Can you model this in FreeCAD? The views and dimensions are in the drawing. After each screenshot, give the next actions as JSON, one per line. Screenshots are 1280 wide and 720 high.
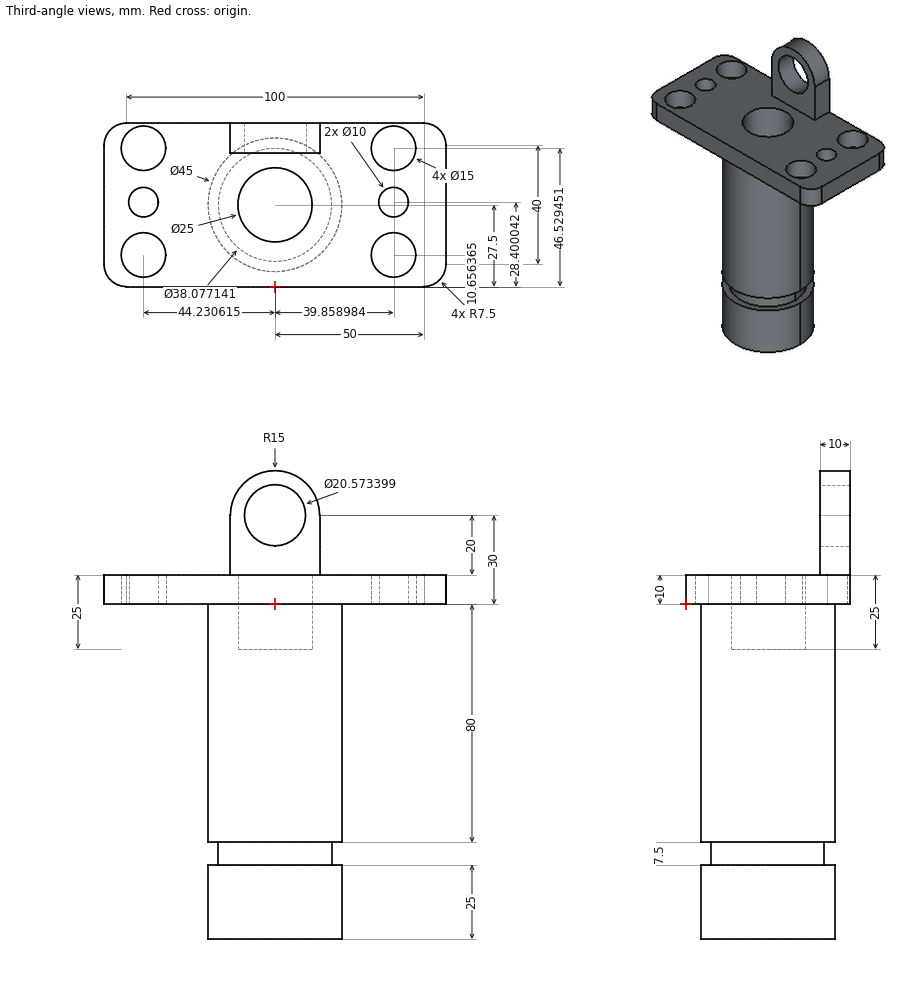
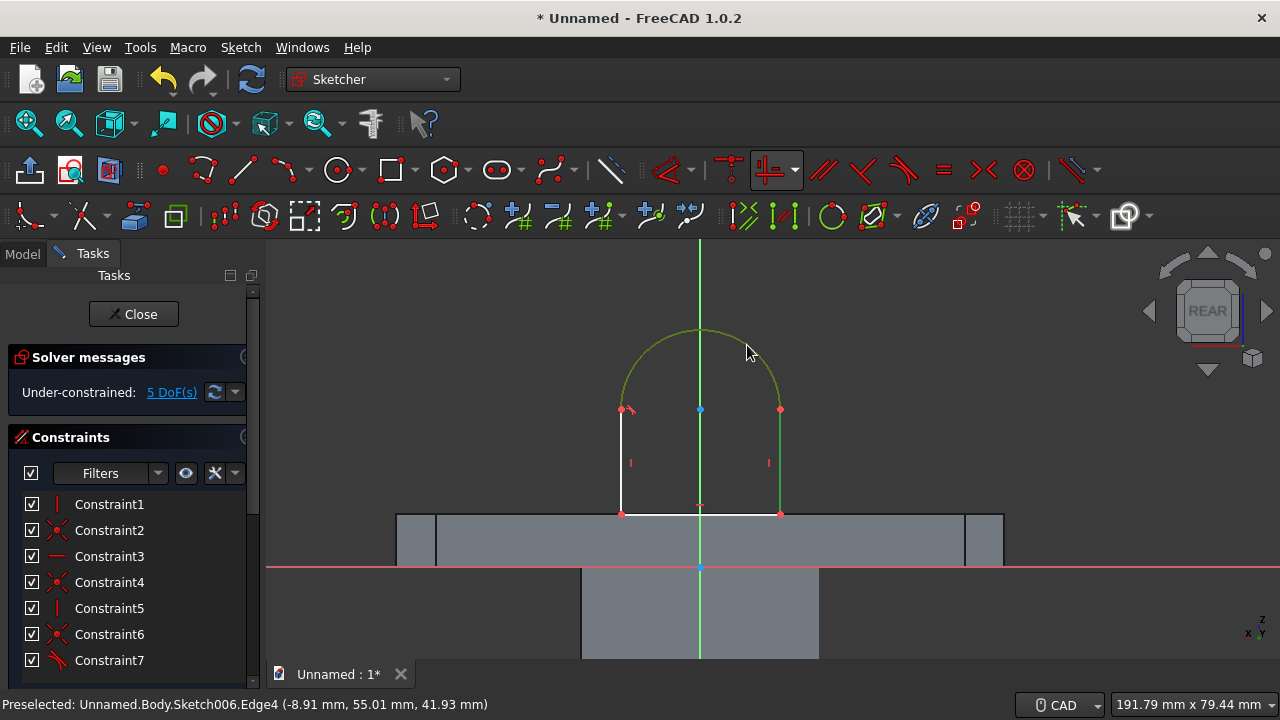
{"action": "left_click", "coordinate": [904, 170]}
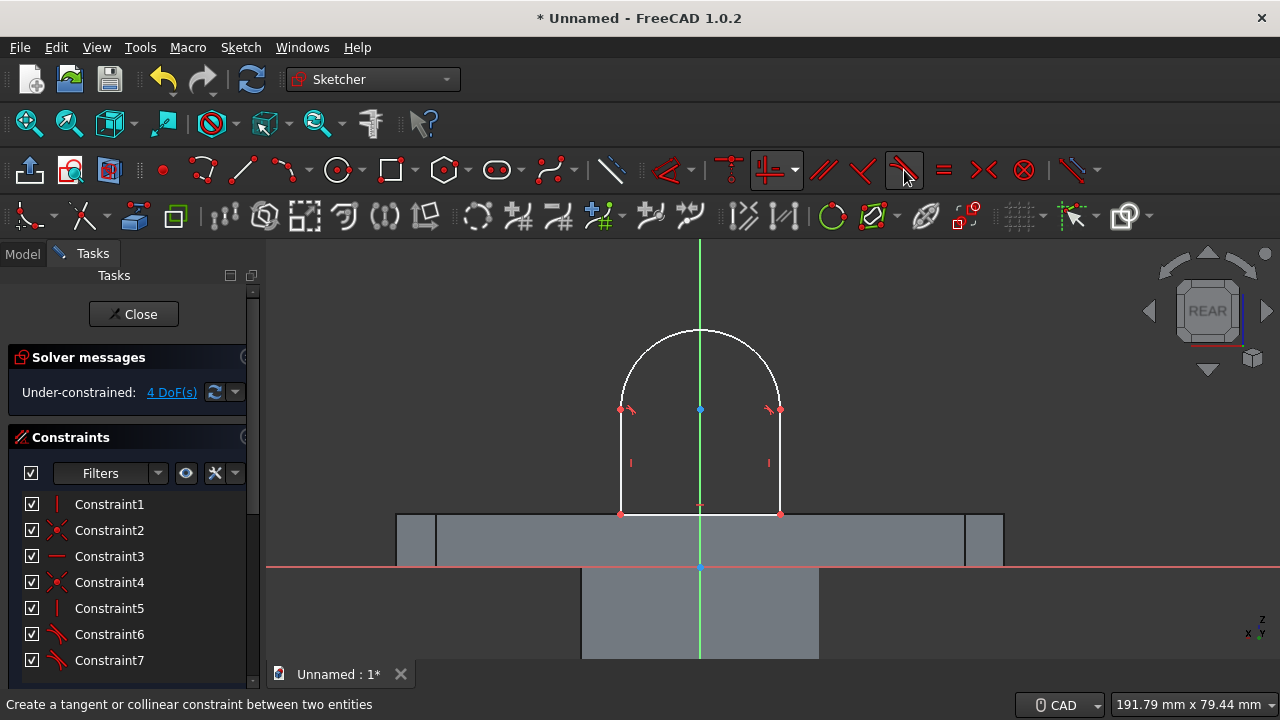
{"action": "left_click", "coordinate": [700, 410]}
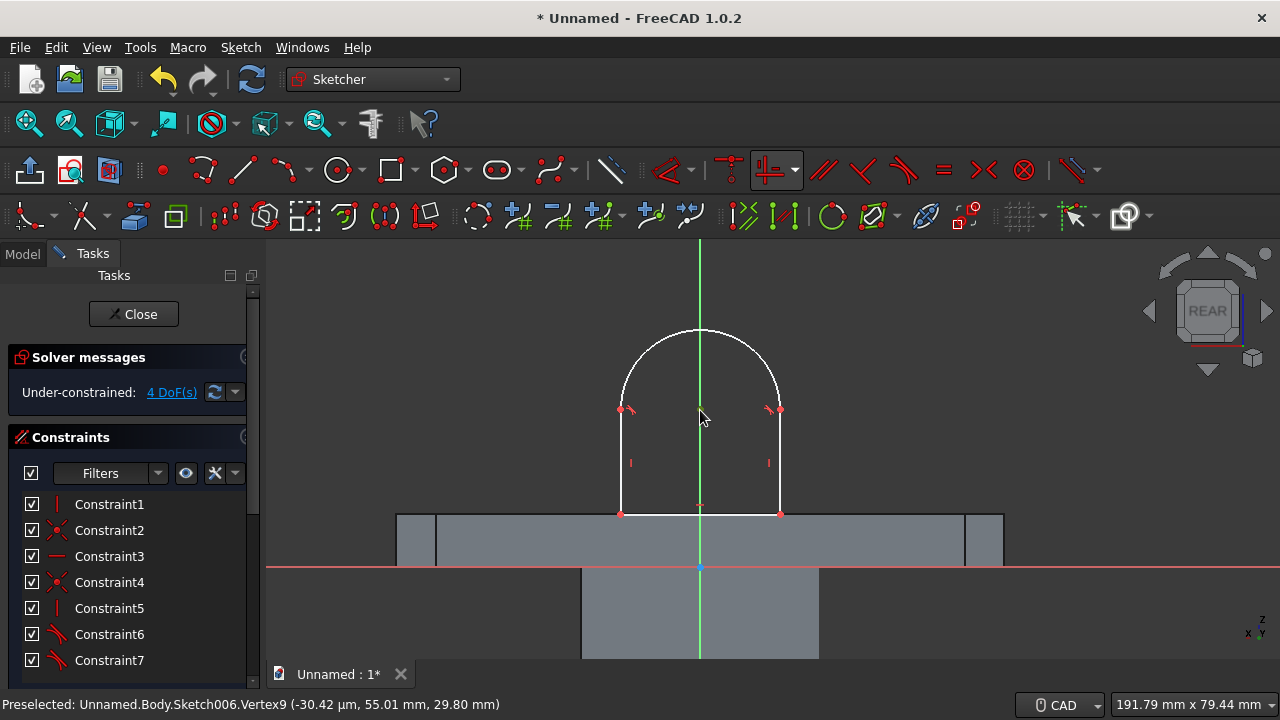
{"action": "left_click", "coordinate": [700, 605]}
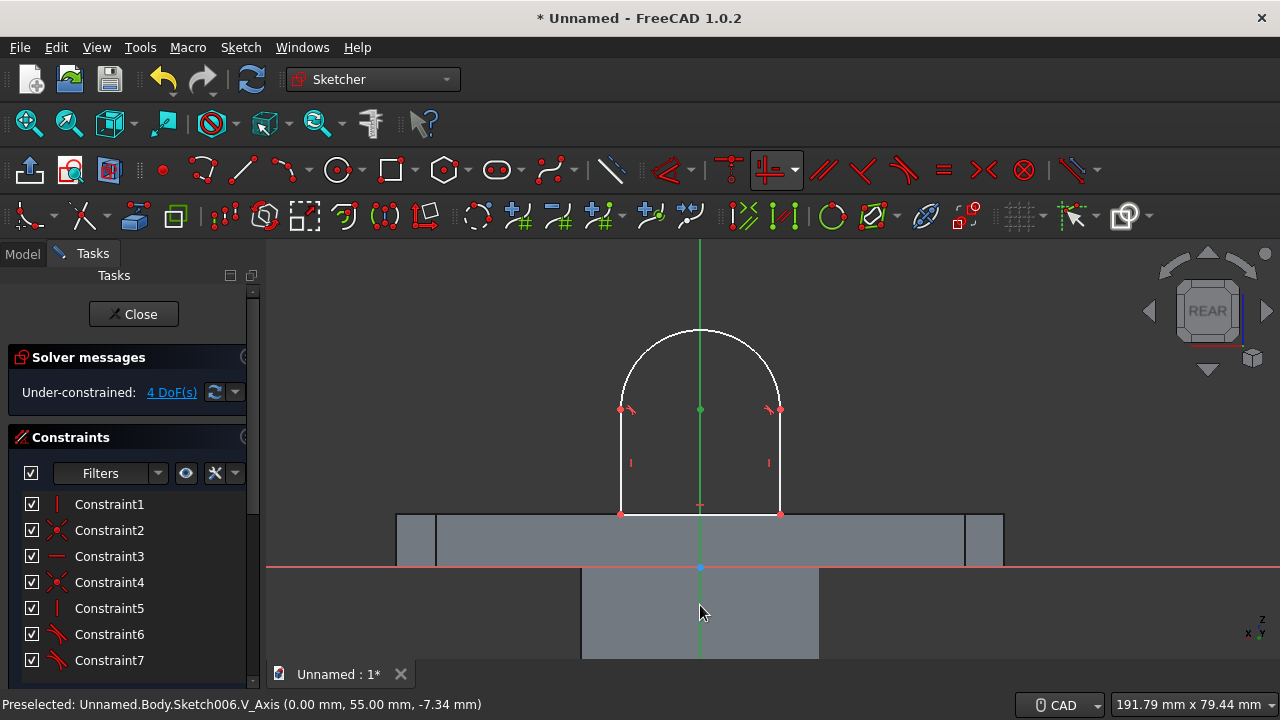
{"action": "left_click", "coordinate": [730, 170]}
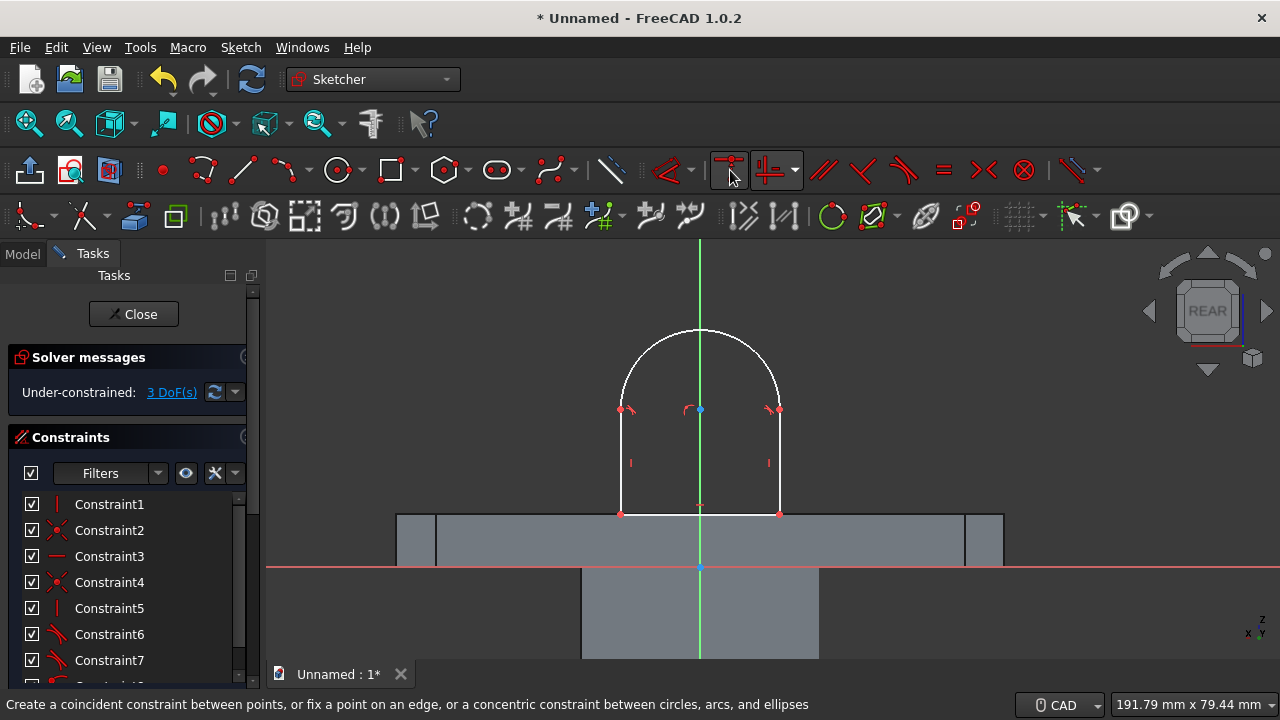
{"action": "left_click", "coordinate": [666, 170]}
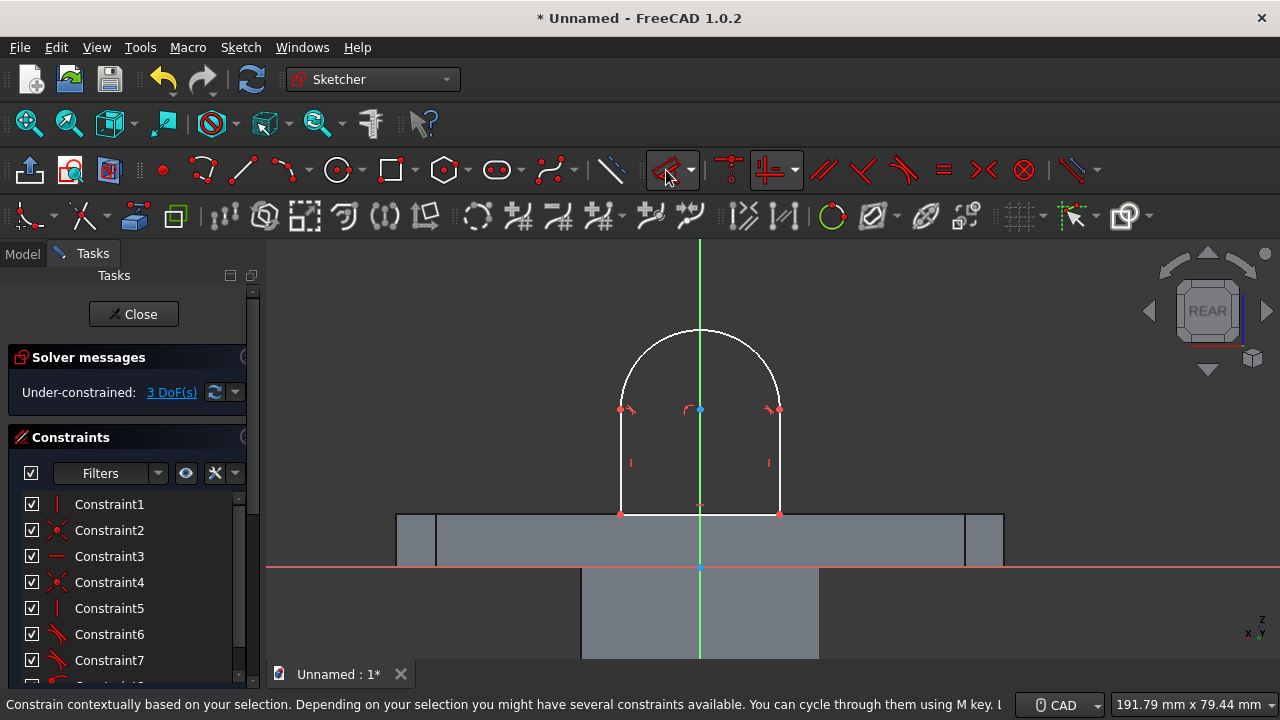
{"action": "left_click", "coordinate": [747, 345]}
{"action": "left_click", "coordinate": [766, 319]}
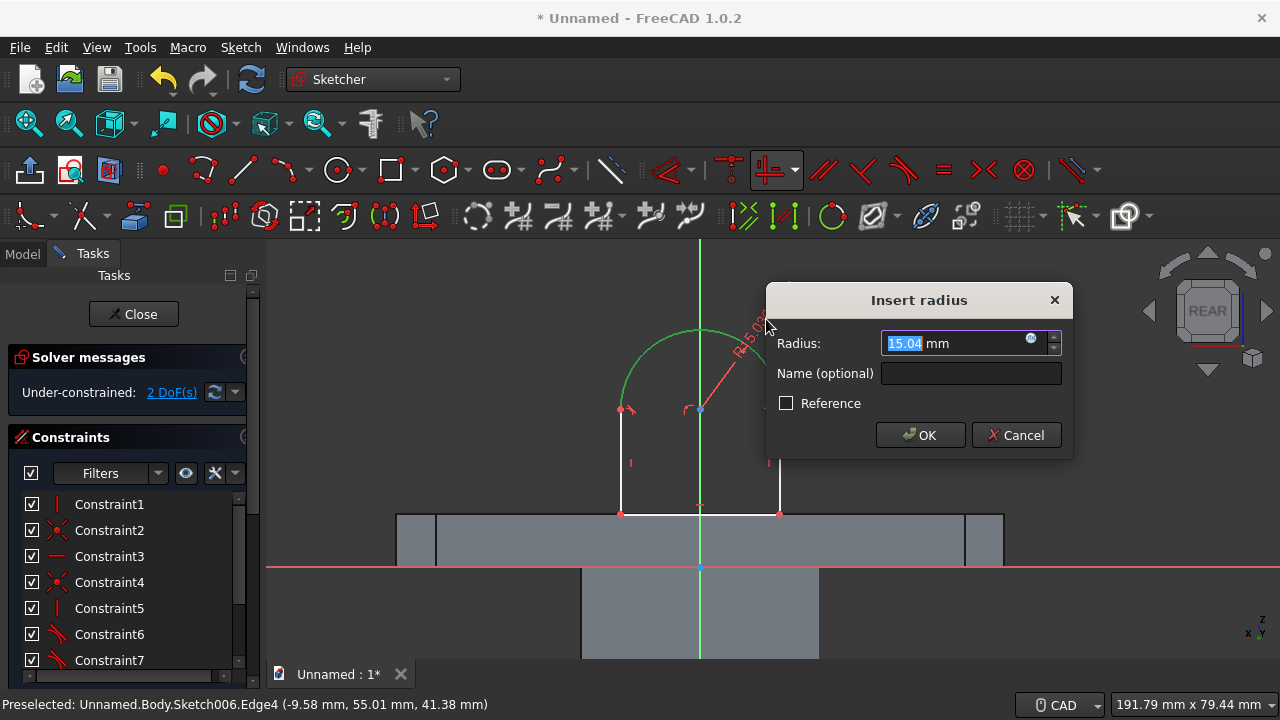
{"action": "type", "text": "15"}
{"action": "key", "text": "Return"}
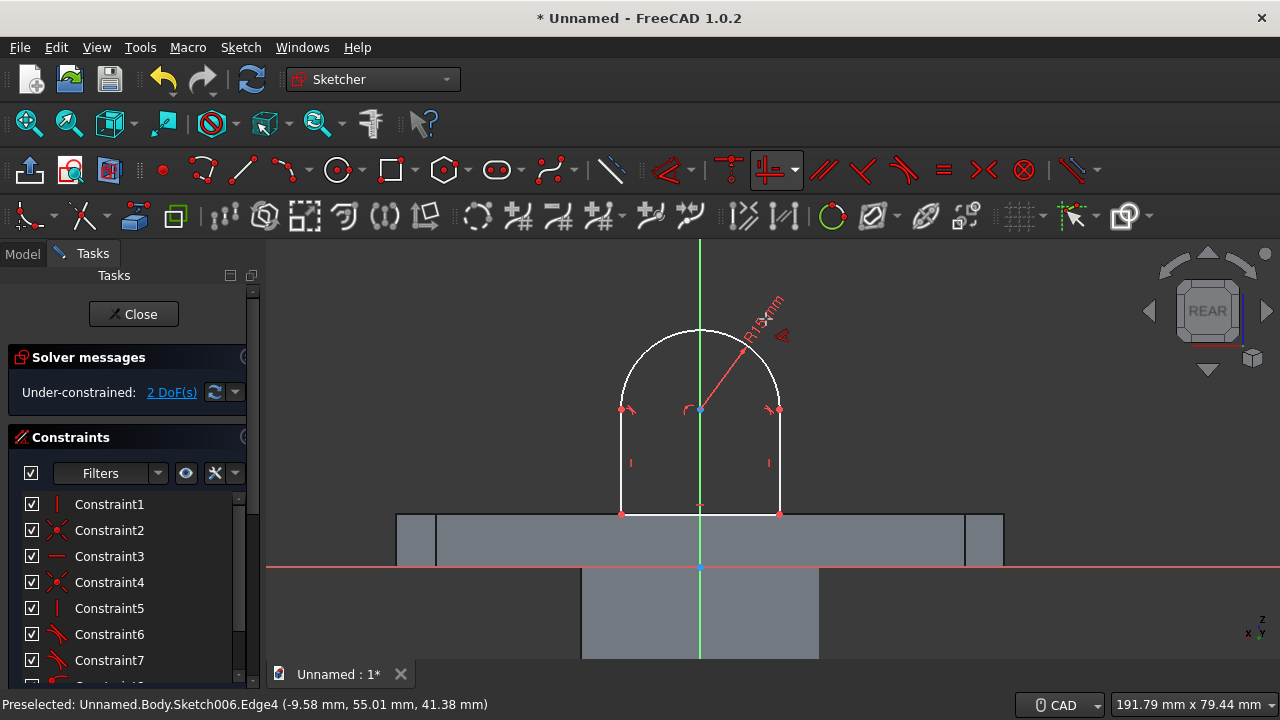
{"action": "left_click", "coordinate": [621, 441]}
{"action": "left_click", "coordinate": [587, 462]}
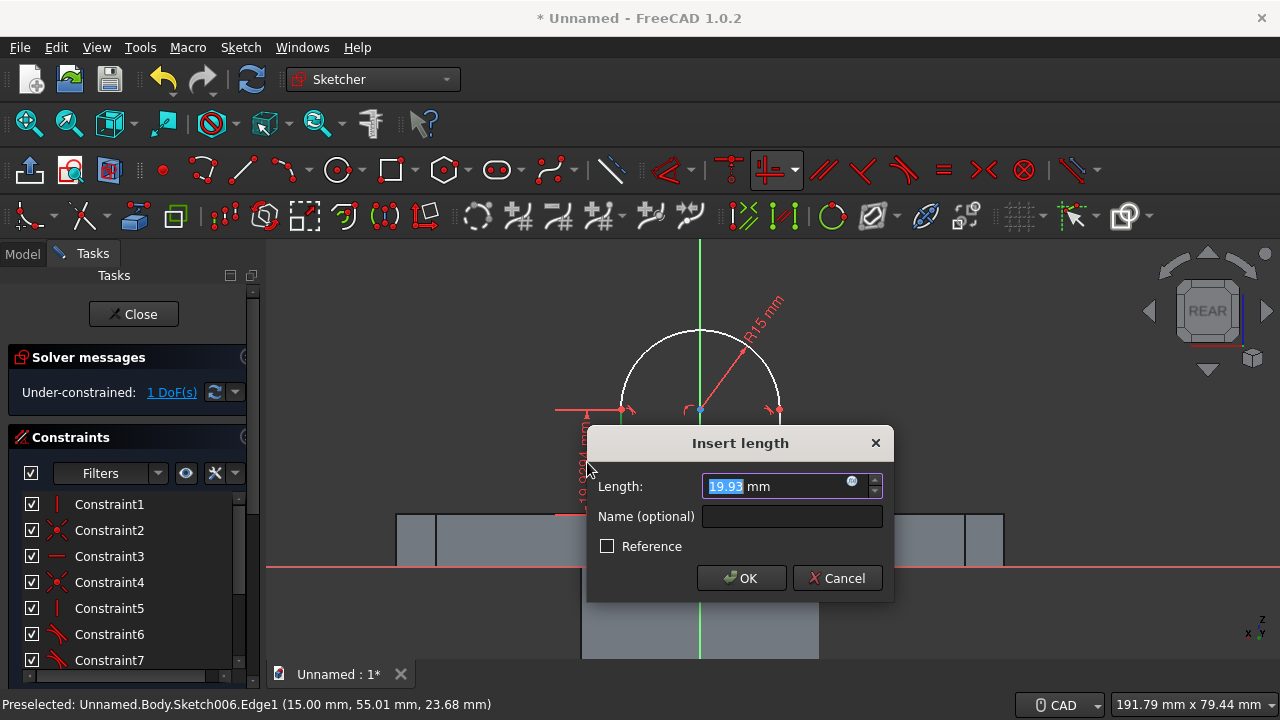
{"action": "type", "text": "20"}
{"action": "key", "text": "Return"}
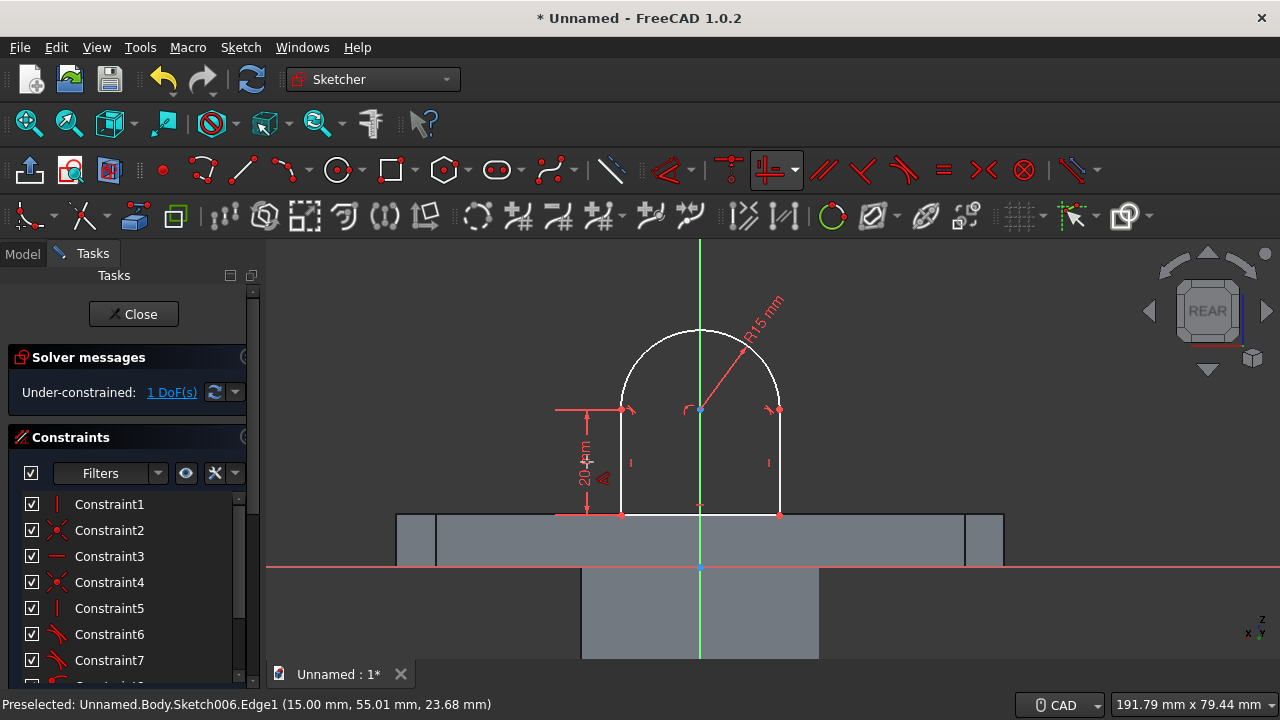
{"action": "left_click", "coordinate": [621, 410]}
{"action": "left_click", "coordinate": [587, 488]}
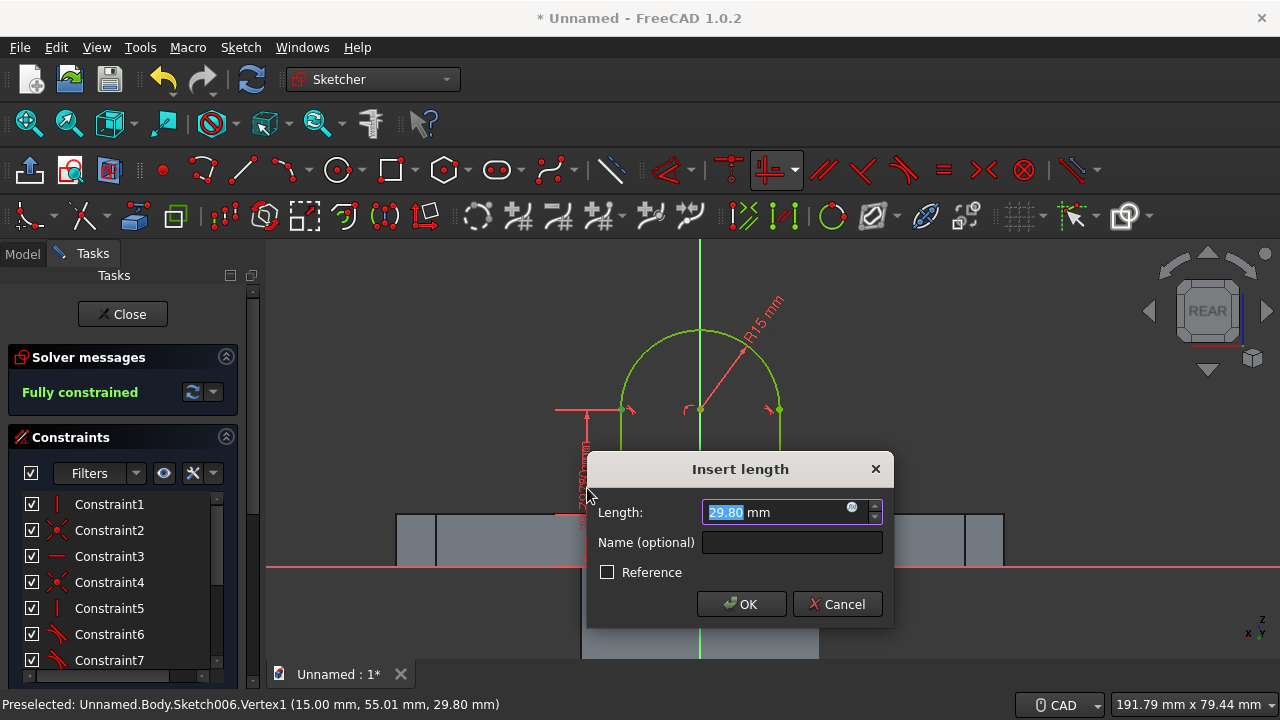
{"action": "type", "text": "30"}
{"action": "key", "text": "Return"}
{"action": "key", "text": "Escape"}